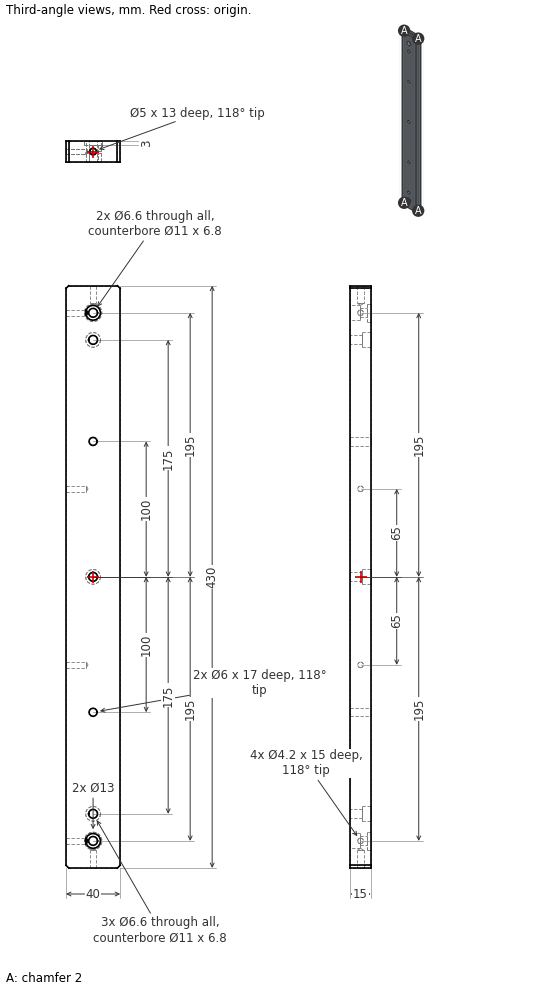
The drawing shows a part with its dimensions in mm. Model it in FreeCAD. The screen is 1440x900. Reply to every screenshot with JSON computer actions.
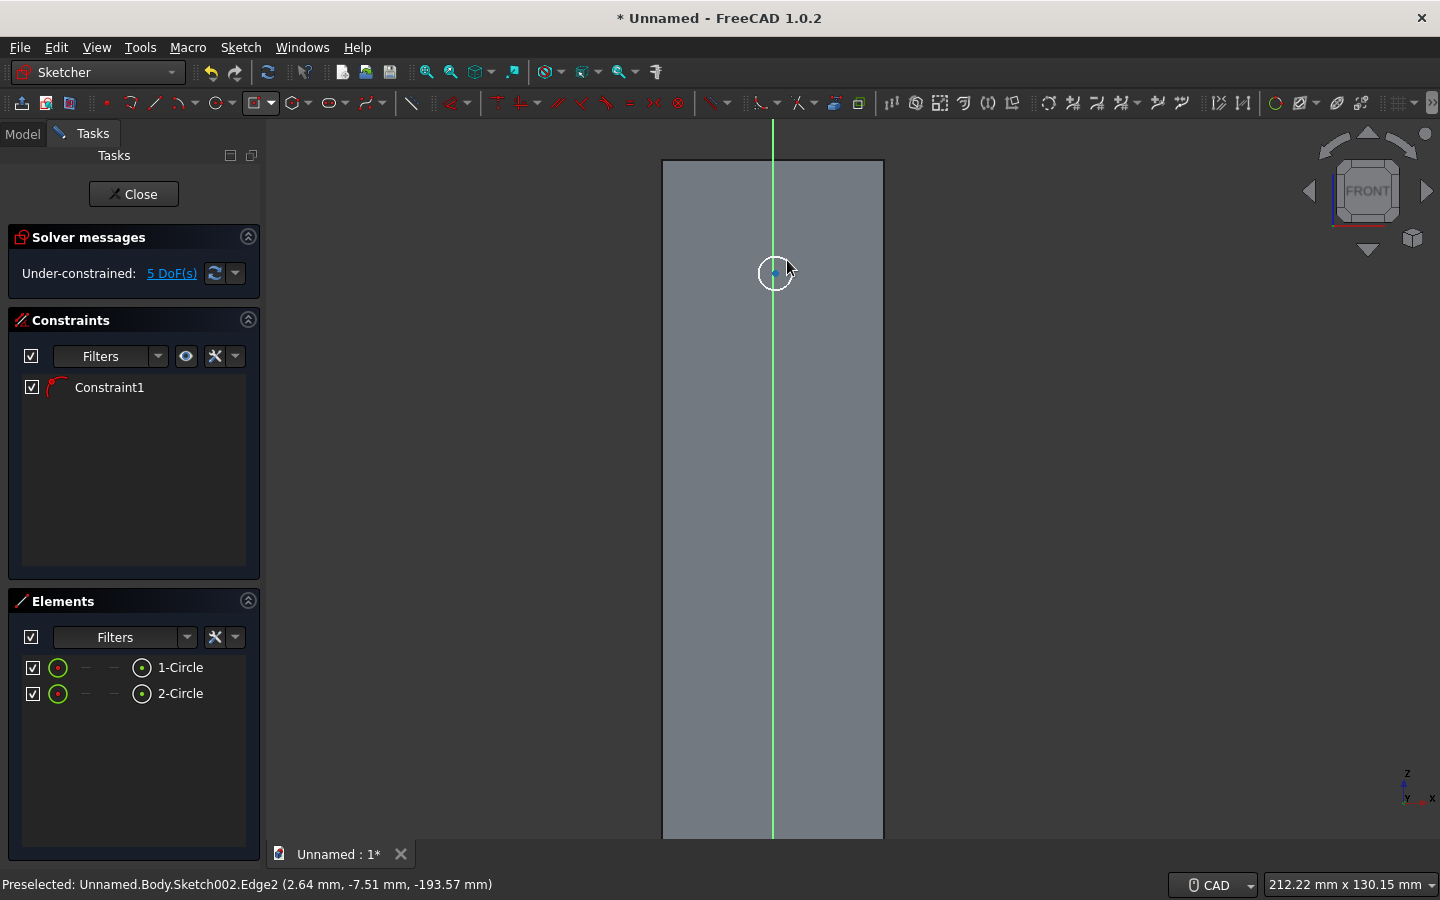
{"action": "left_click", "coordinate": [787, 262]}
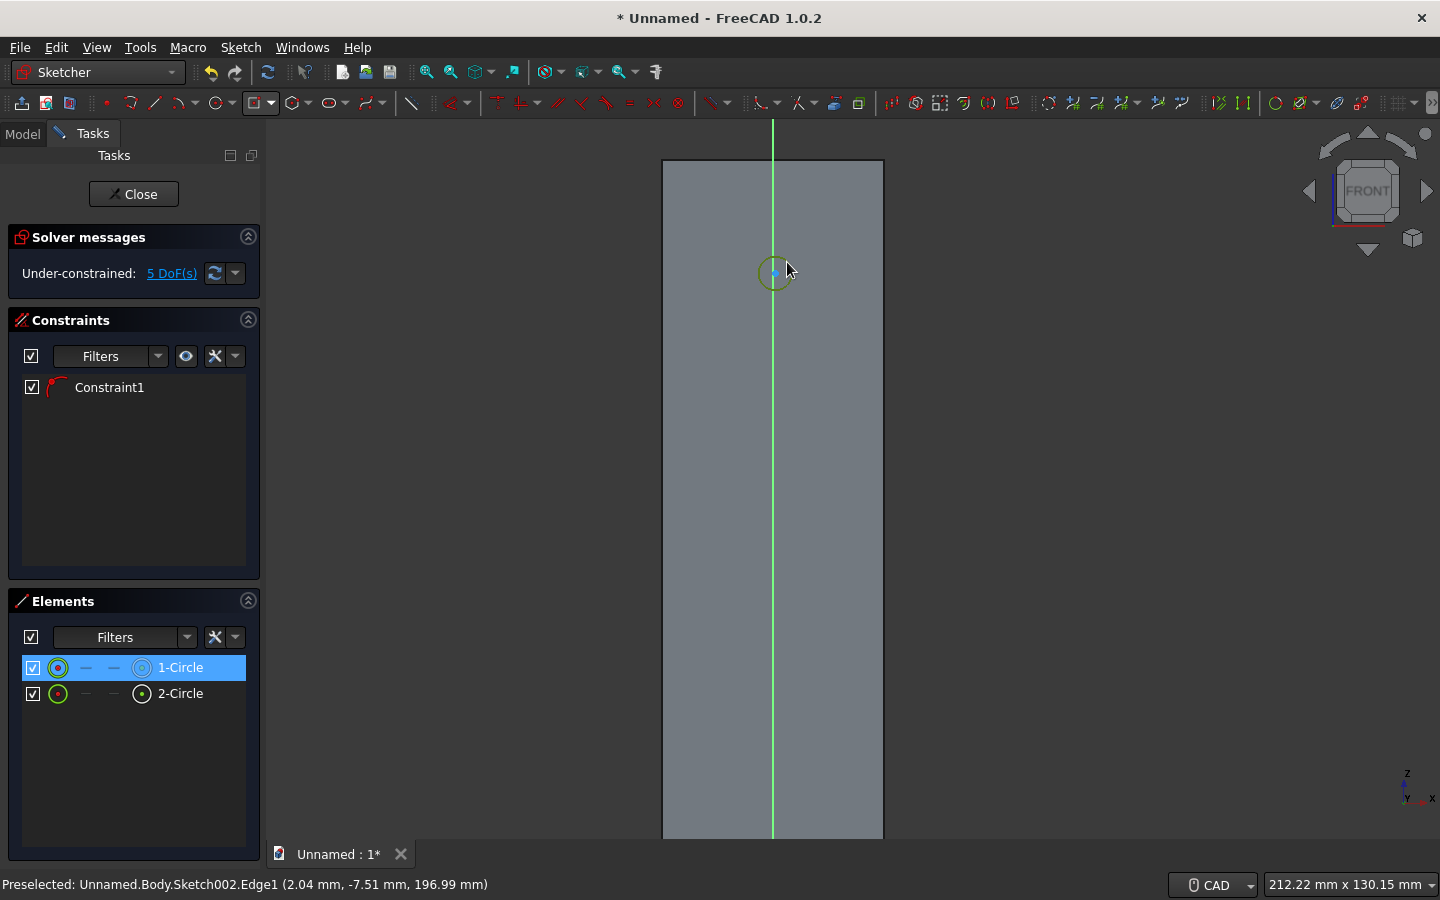
{"action": "scroll", "coordinate": [787, 259], "scroll_direction": "down", "scroll_amount": 8}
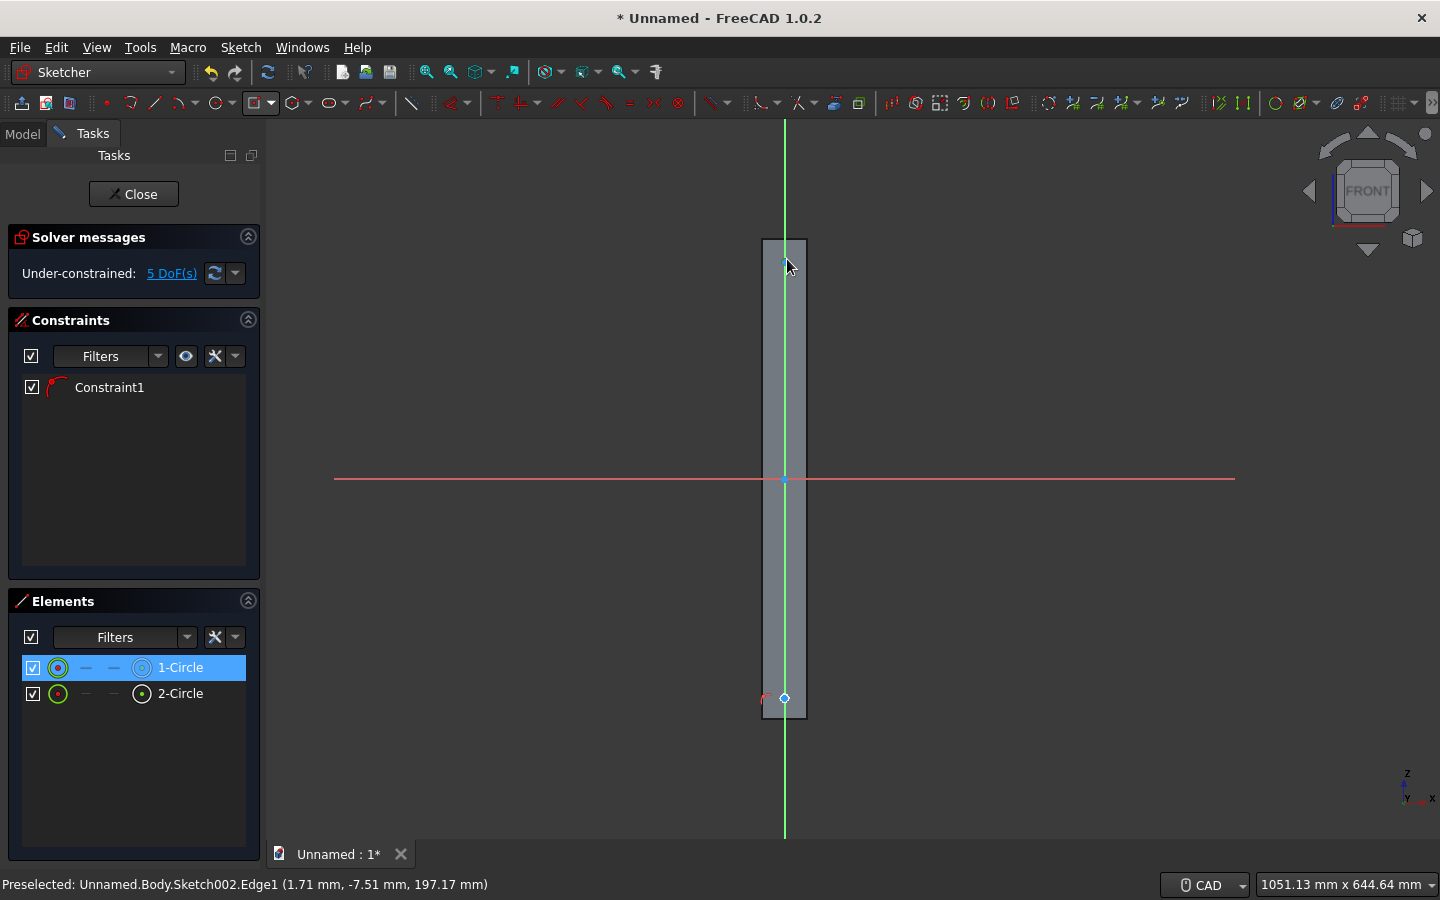
{"action": "scroll", "coordinate": [787, 695], "scroll_direction": "up", "scroll_amount": 8}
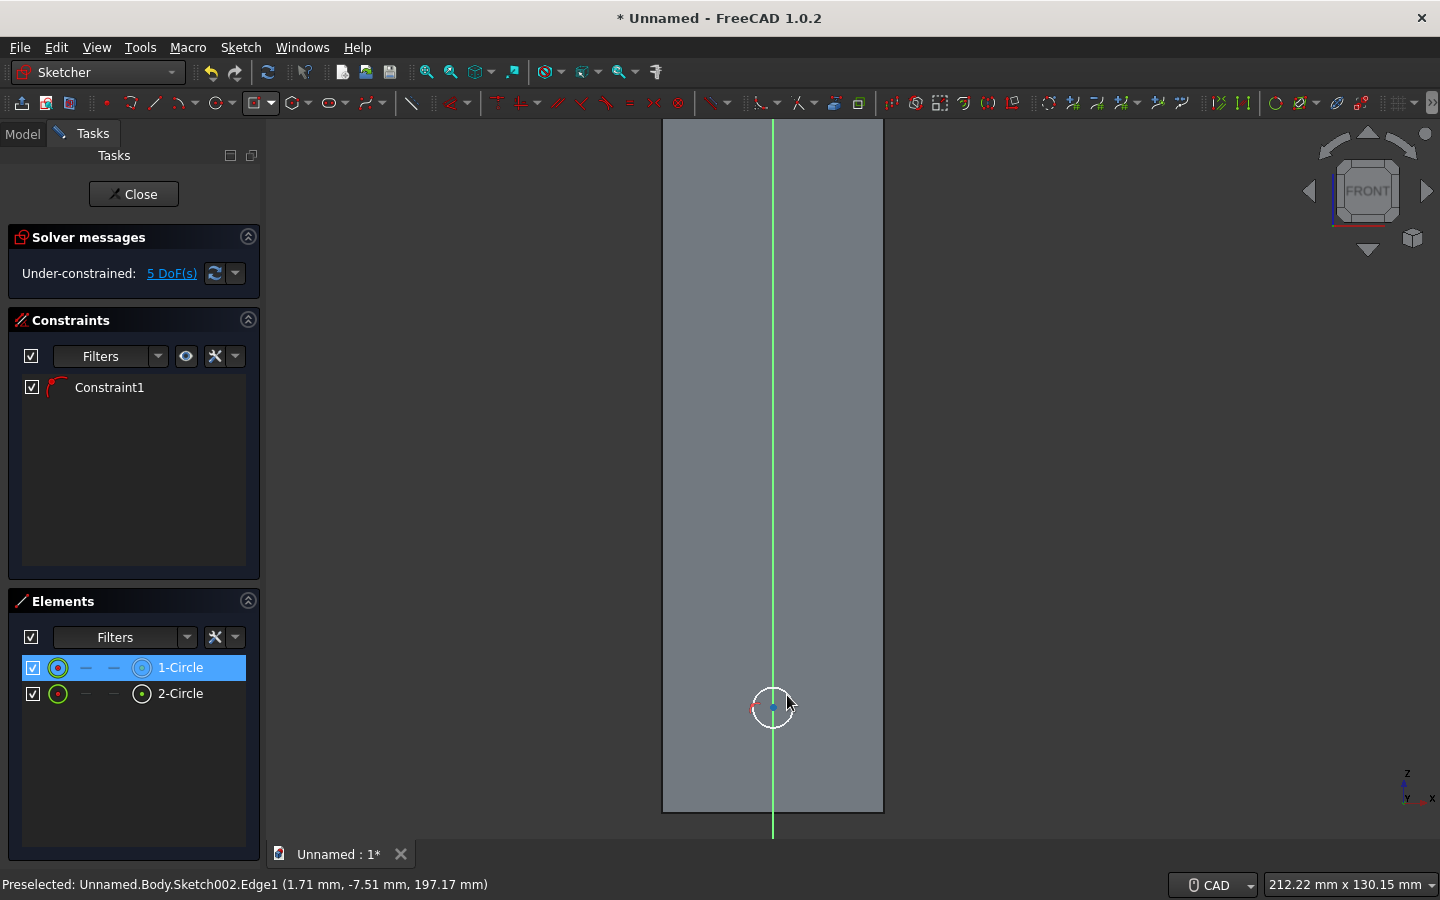
{"action": "left_click", "coordinate": [787, 693]}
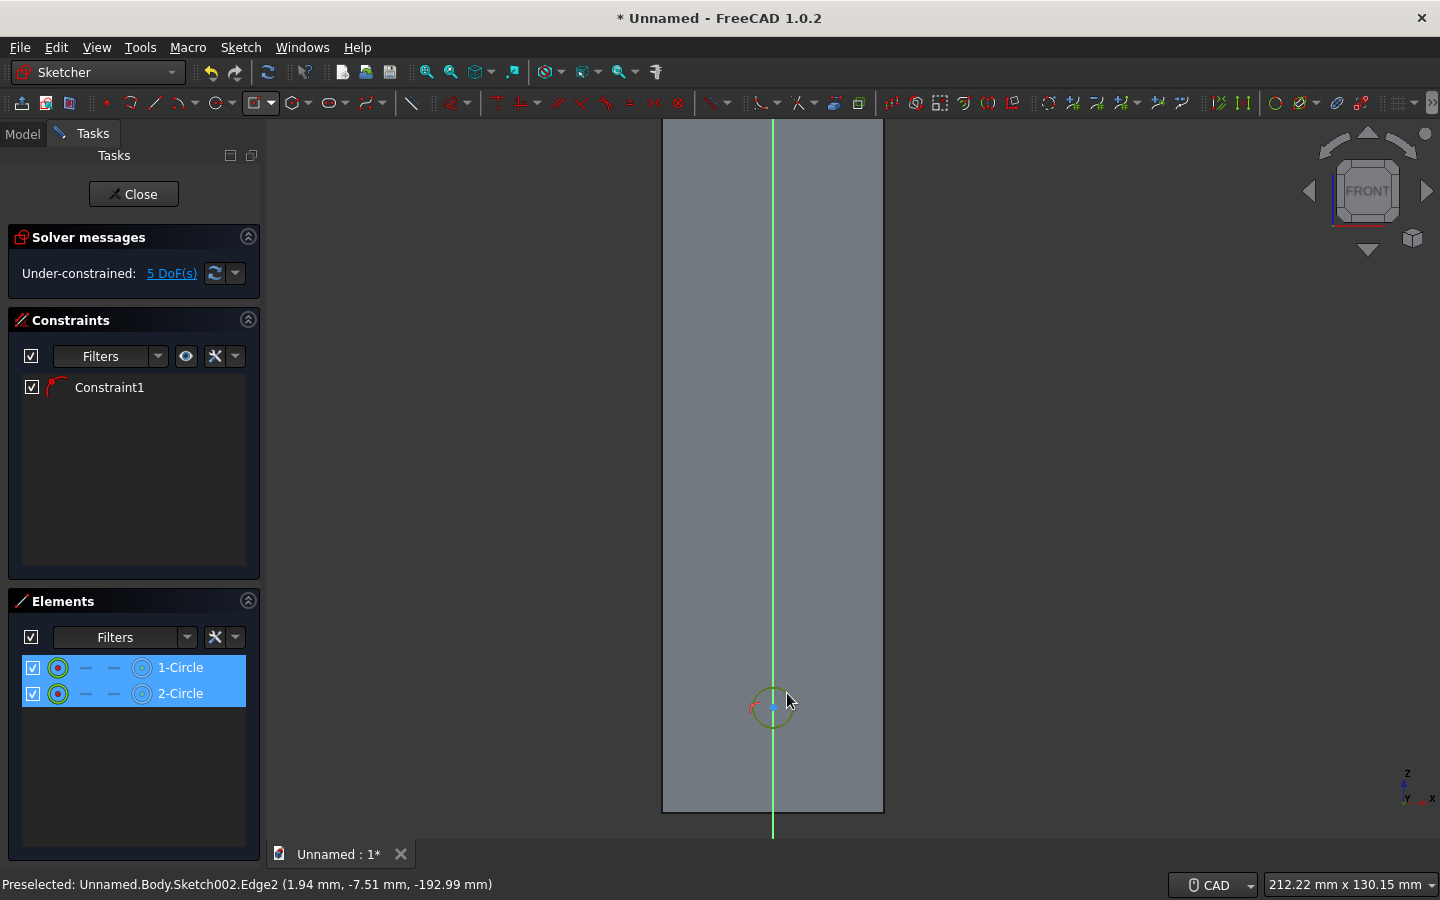
{"action": "key", "text": "e"}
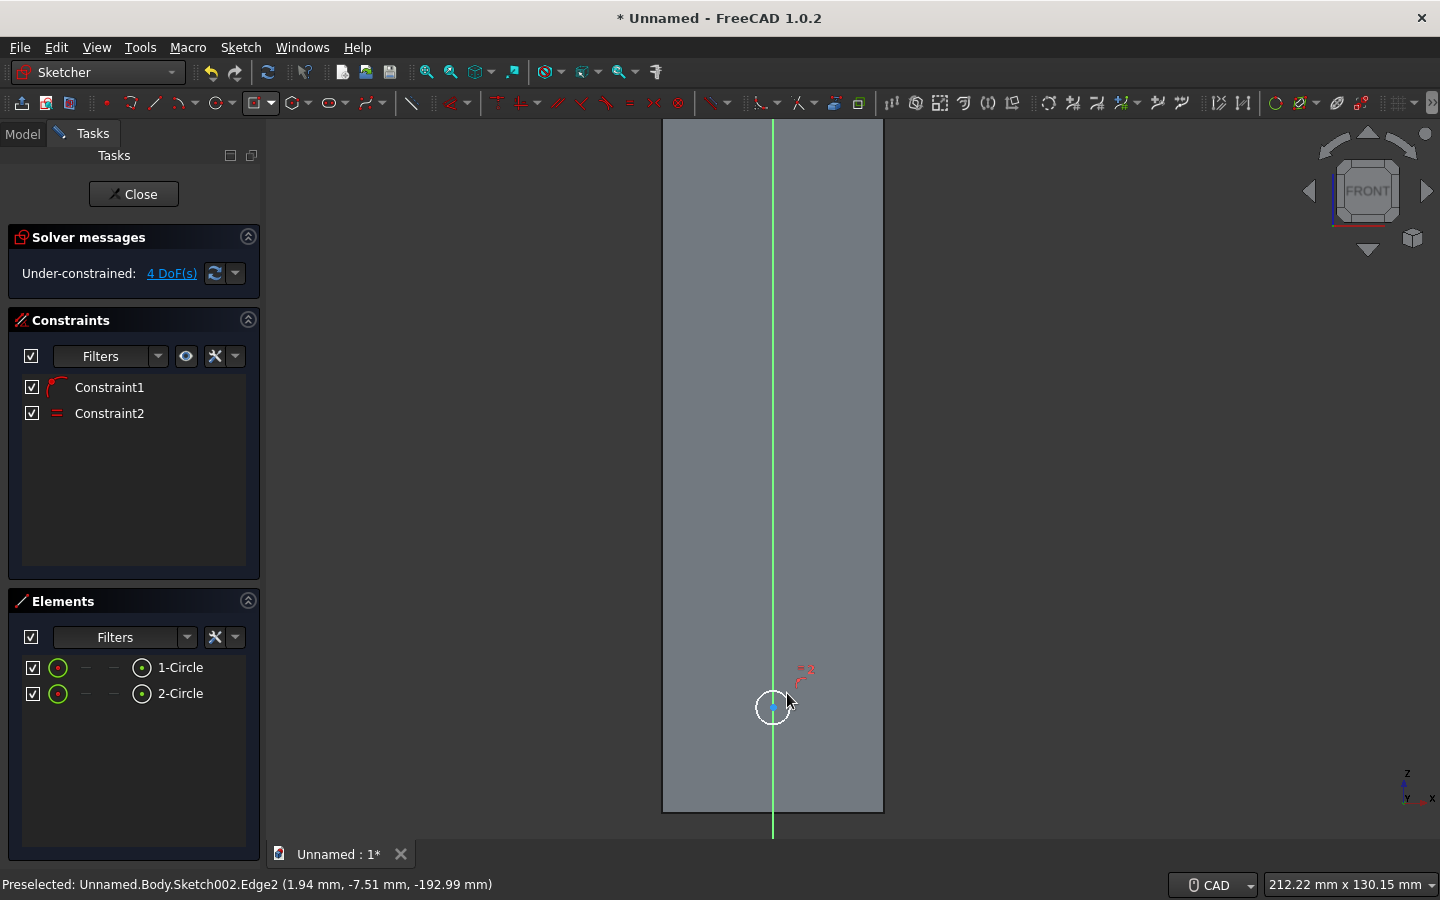
{"action": "scroll", "coordinate": [787, 696], "scroll_direction": "down", "scroll_amount": 8}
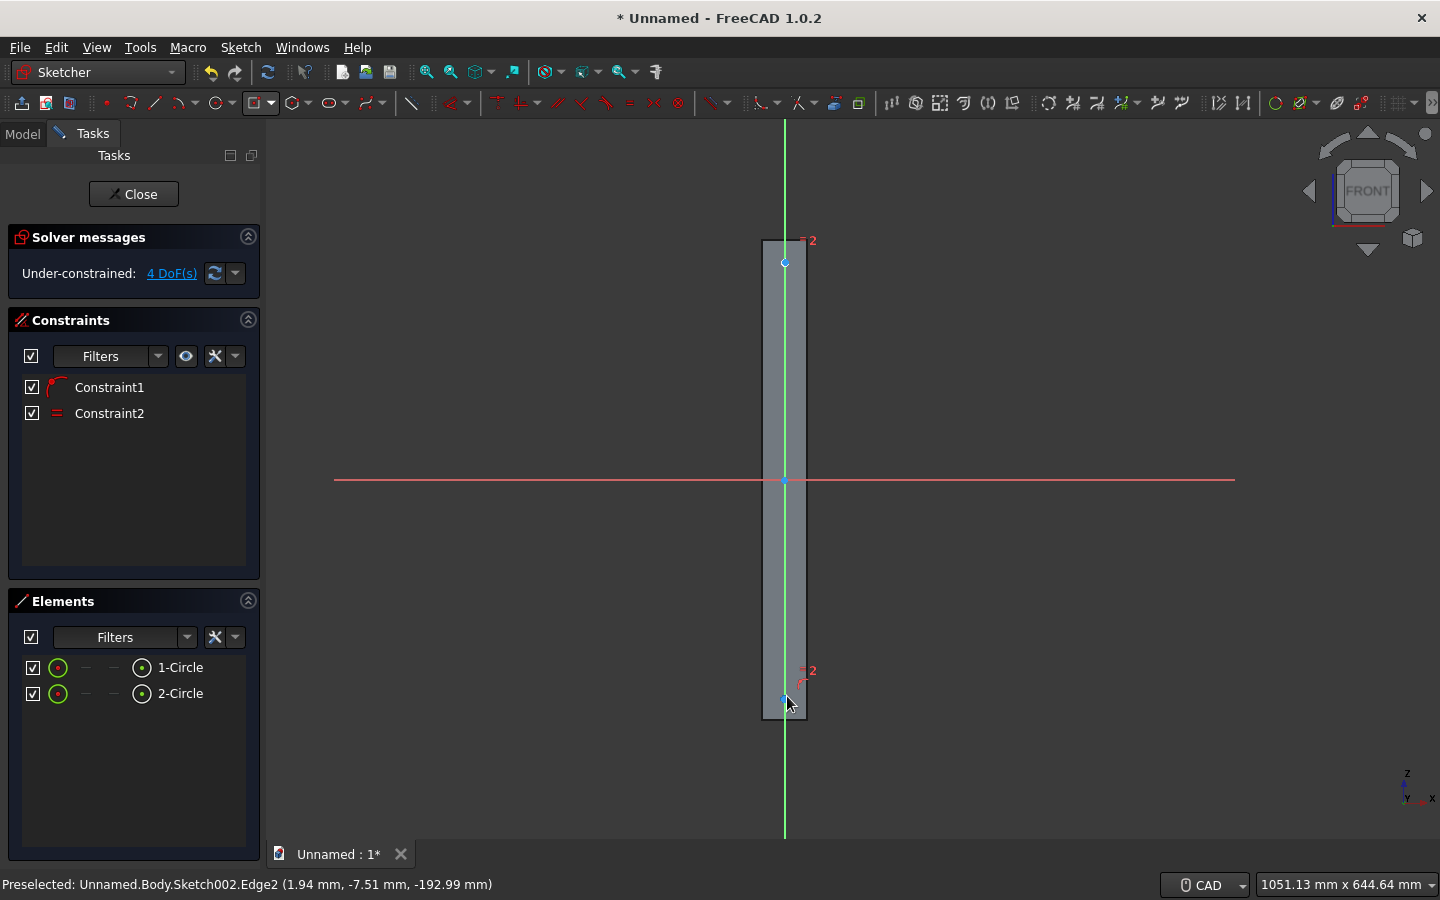
{"action": "left_click", "coordinate": [785, 263]}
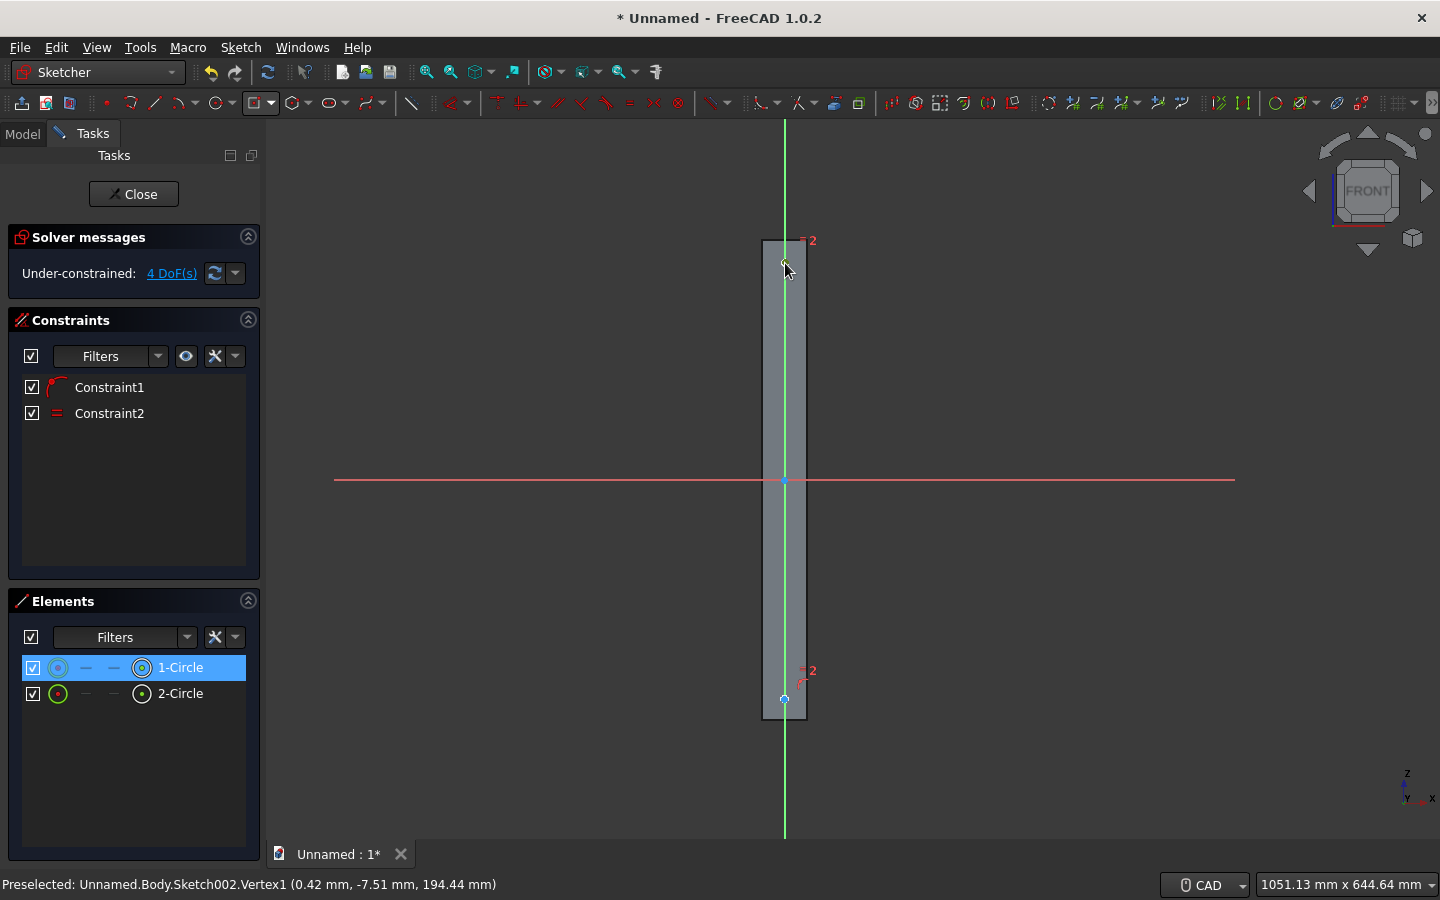
{"action": "left_click", "coordinate": [785, 764]}